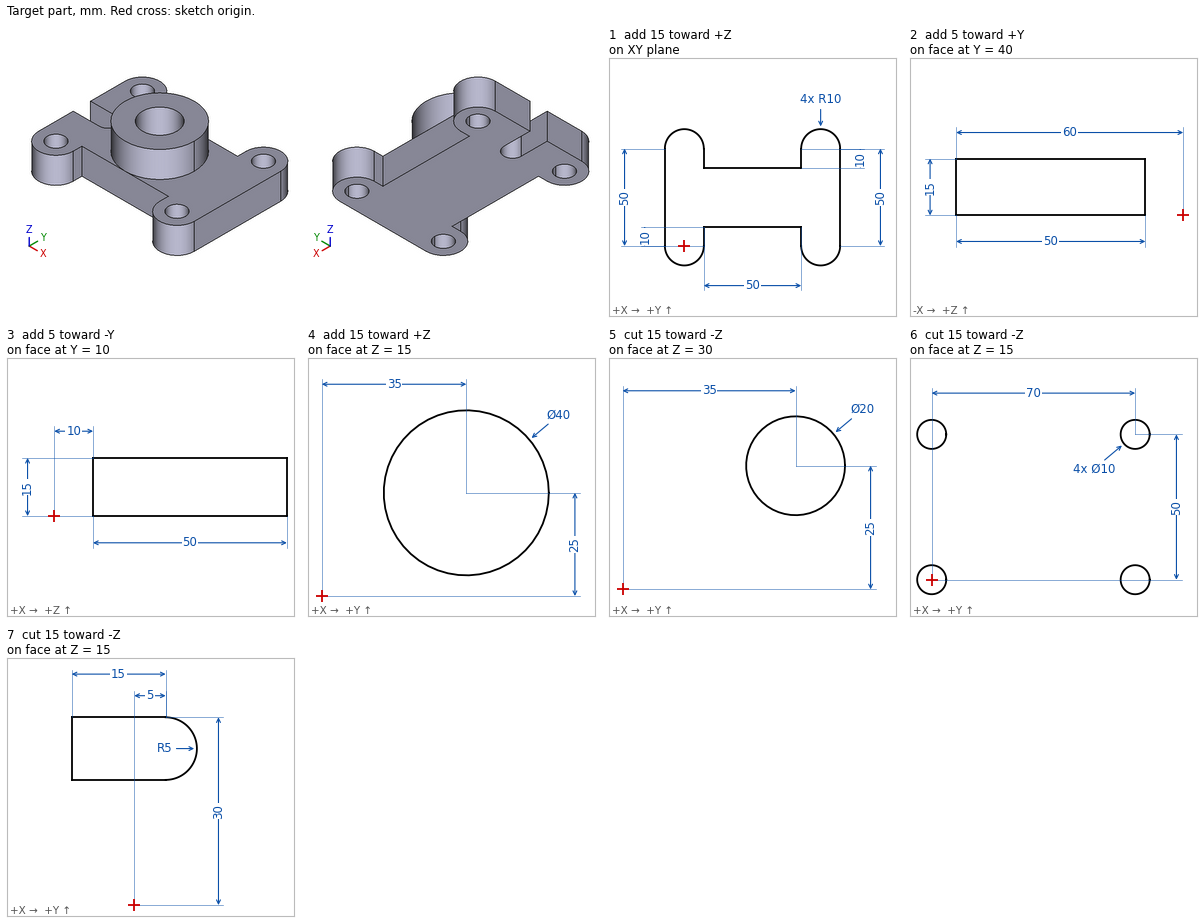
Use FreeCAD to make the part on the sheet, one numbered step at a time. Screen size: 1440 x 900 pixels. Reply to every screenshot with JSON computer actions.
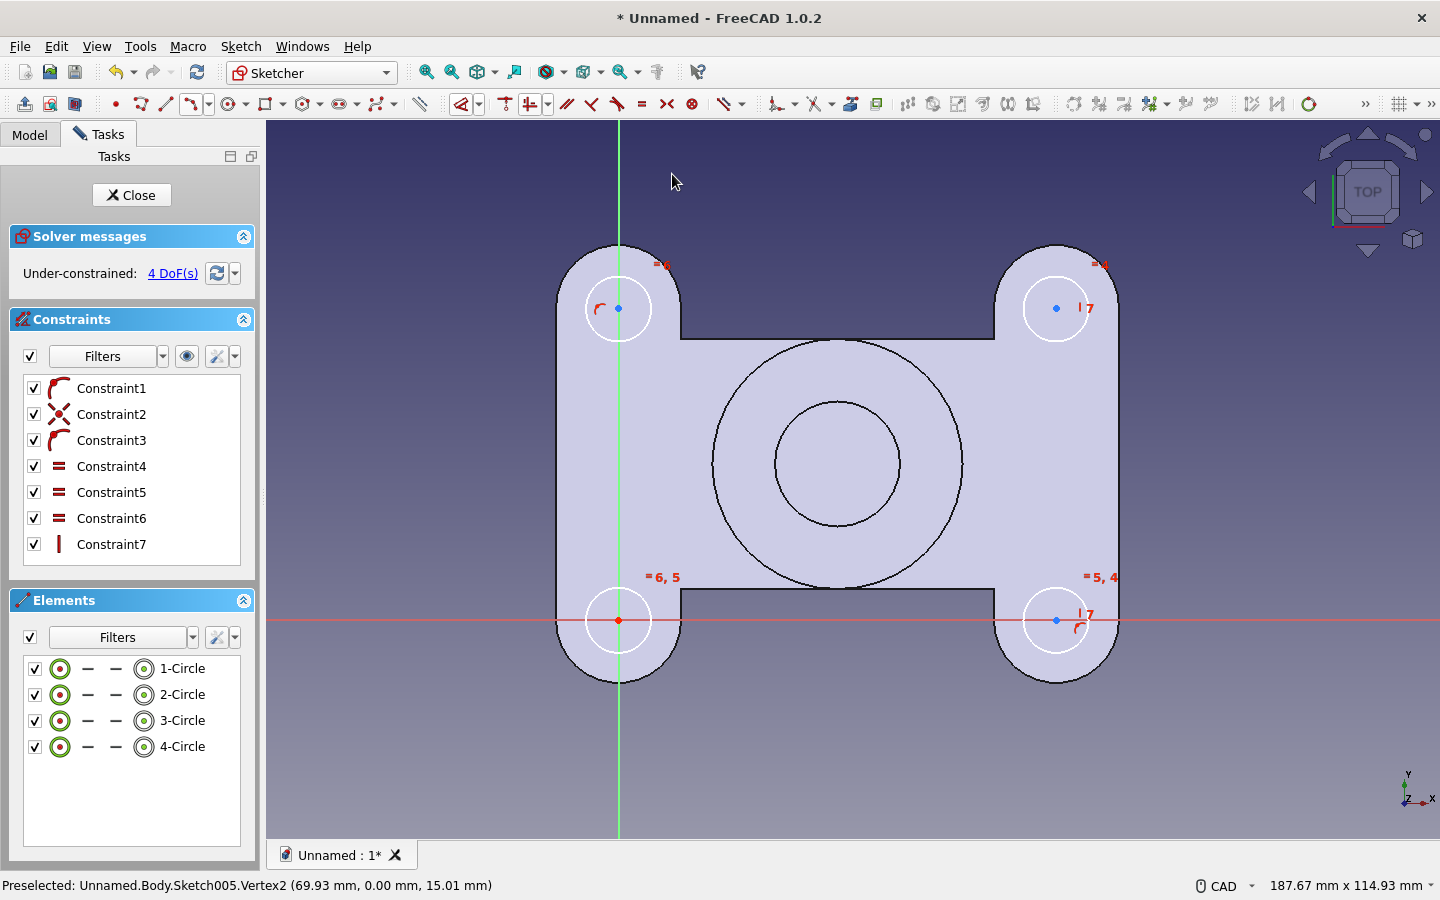
{"action": "left_click", "coordinate": [1056, 309]}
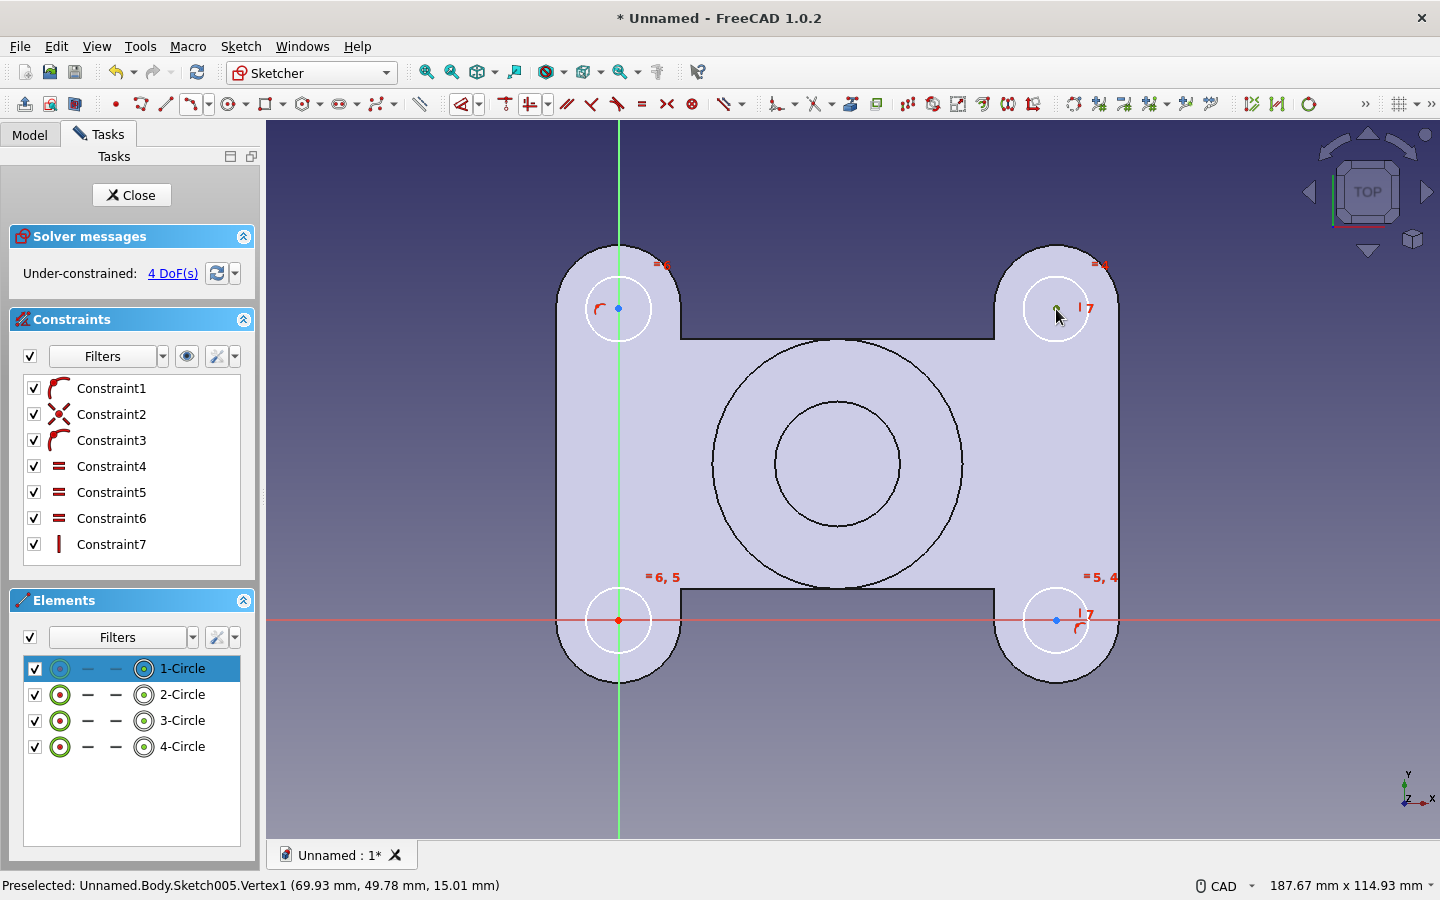
{"action": "left_click", "coordinate": [619, 309]}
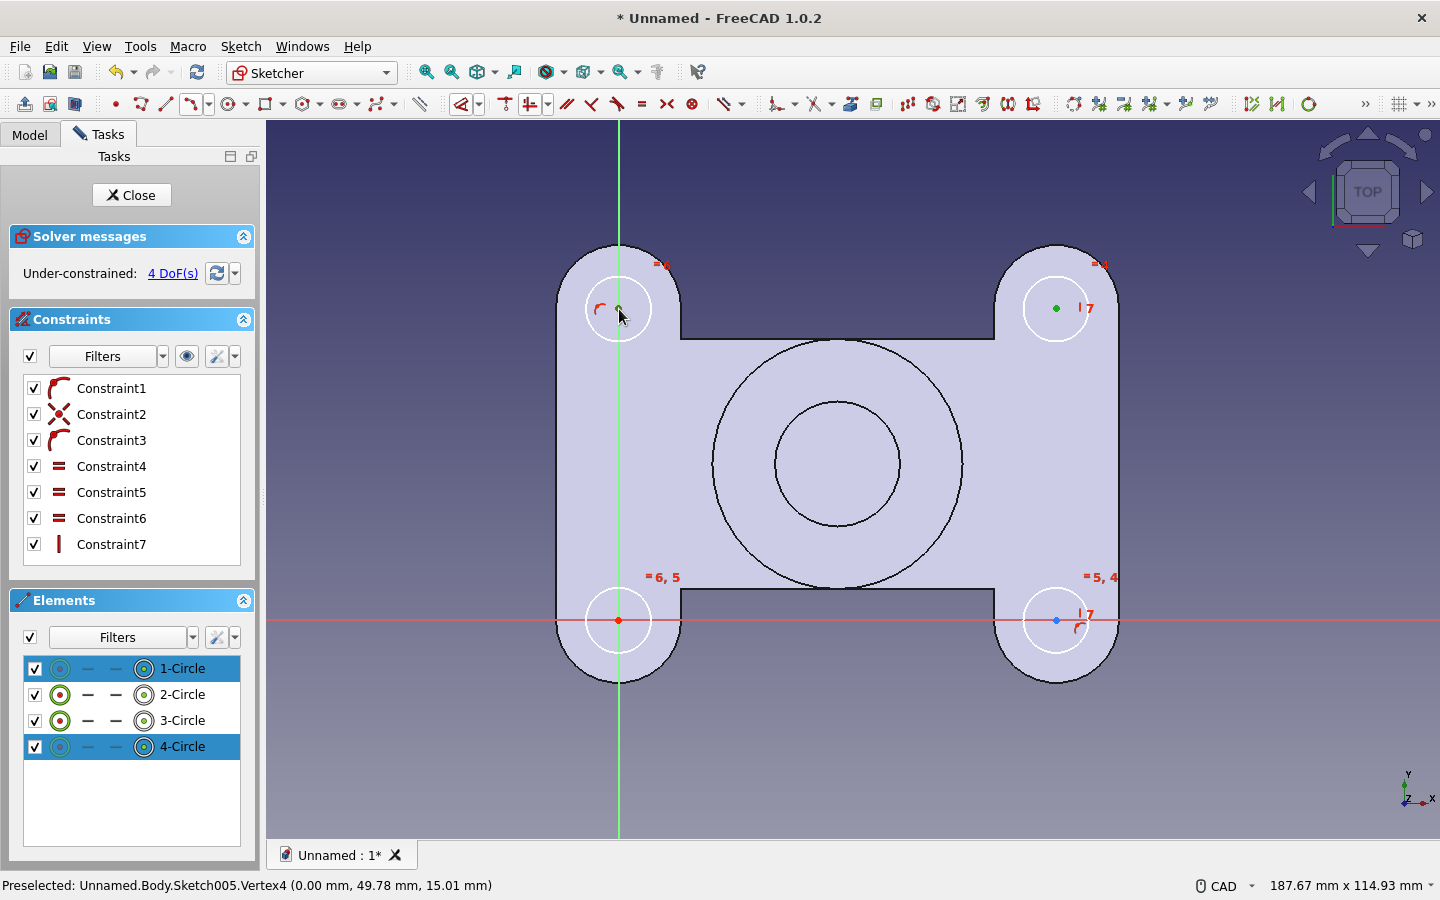
{"action": "left_click", "coordinate": [548, 104]}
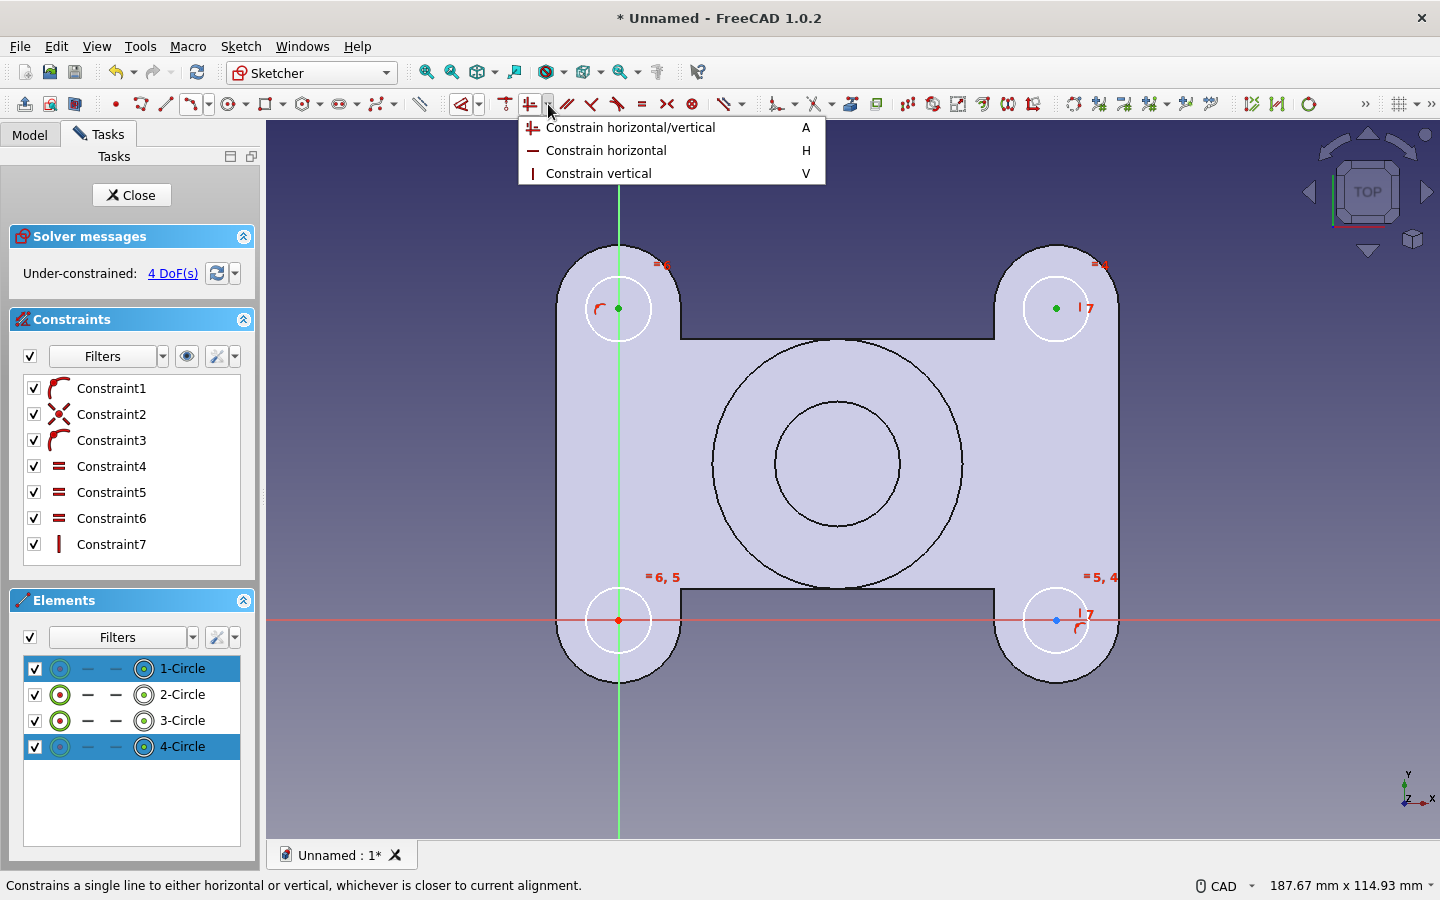
{"action": "left_click", "coordinate": [672, 150]}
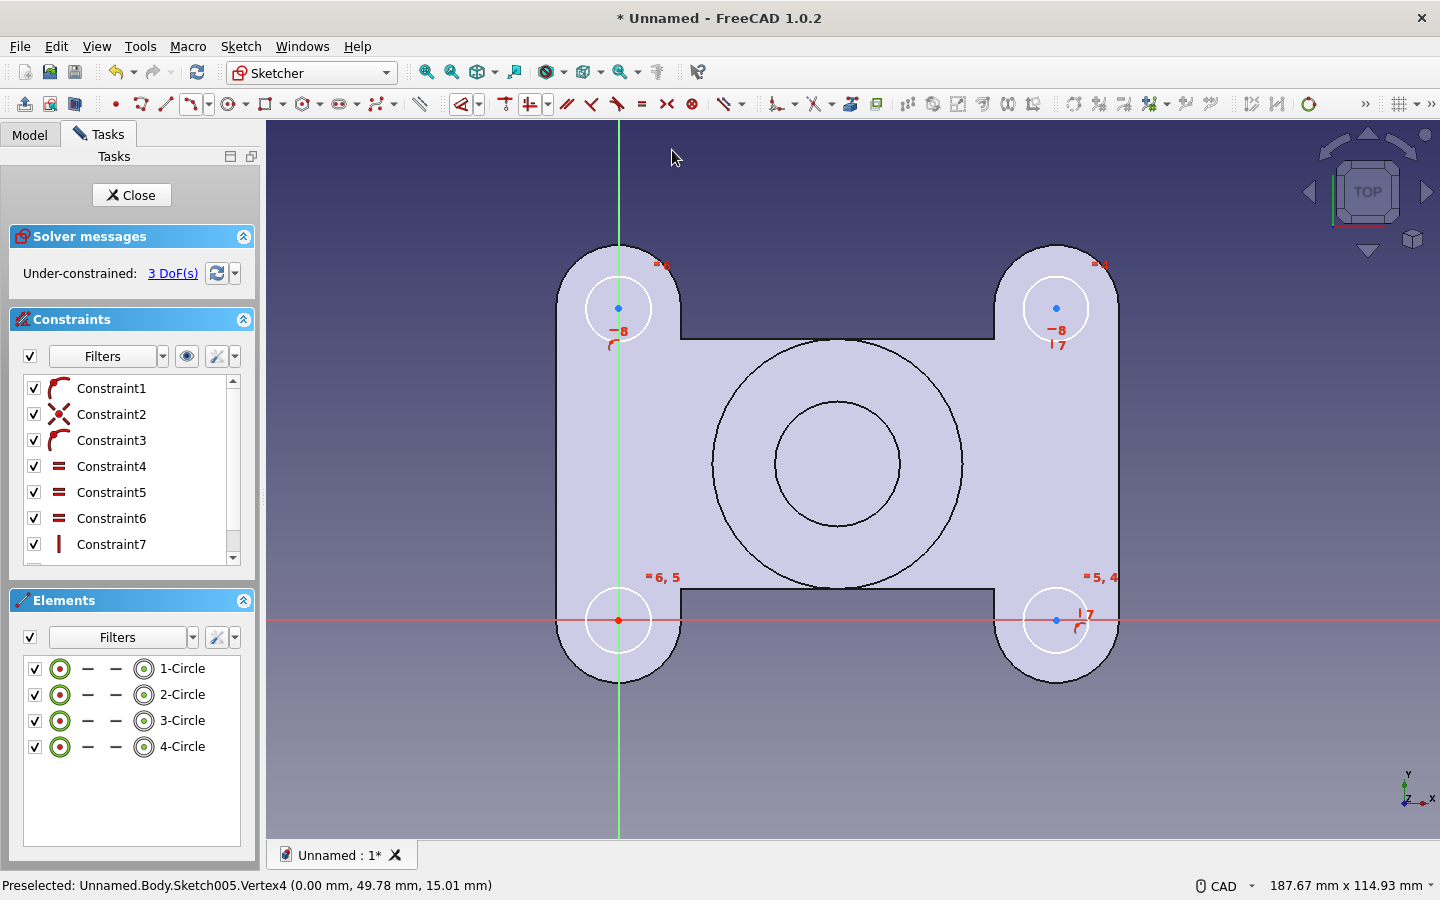
{"action": "left_click", "coordinate": [1079, 286]}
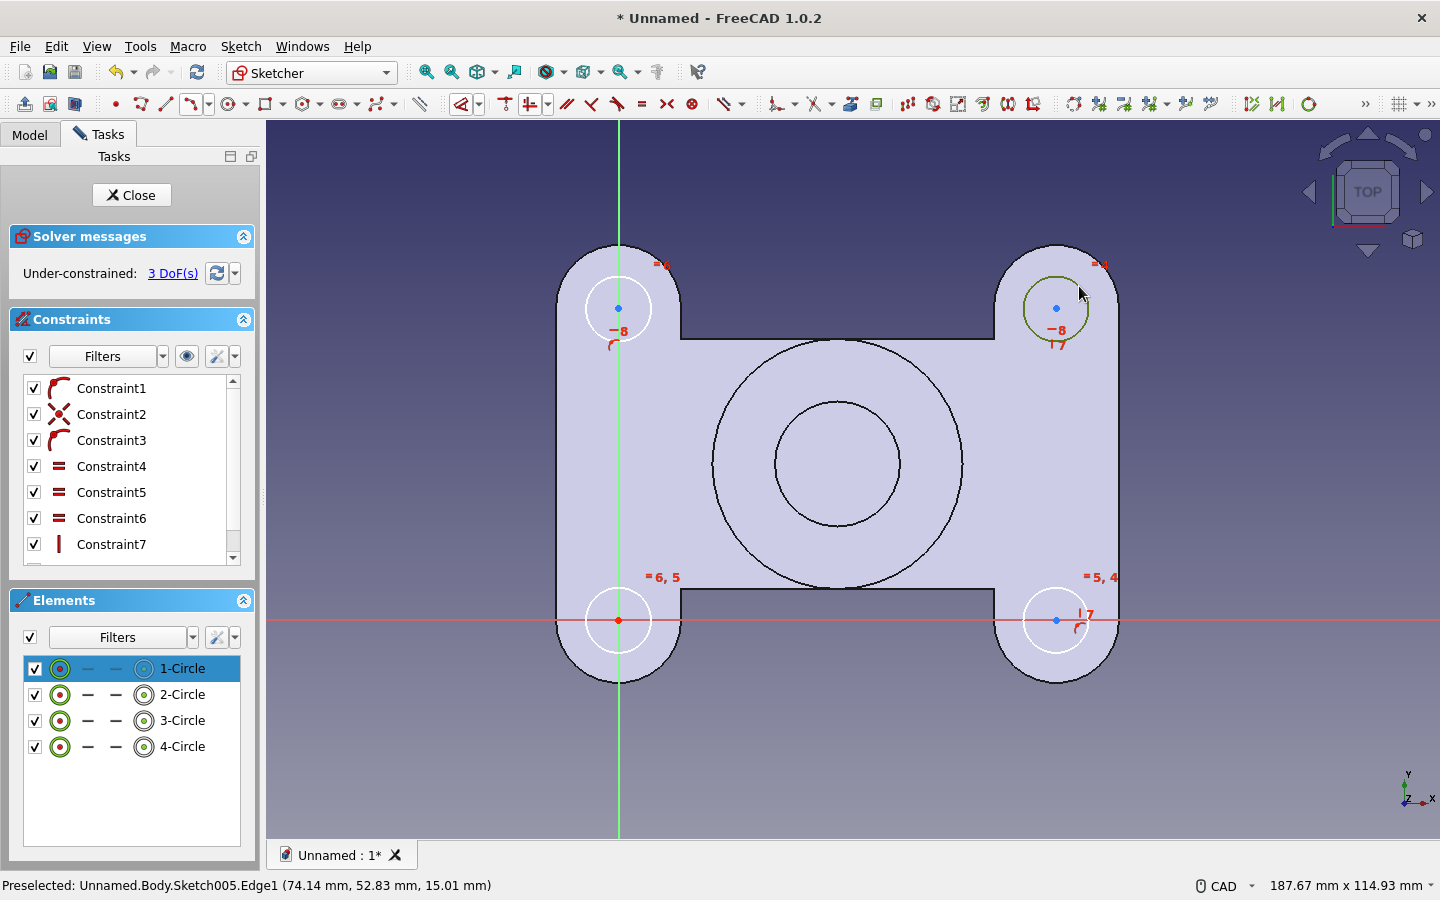
{"action": "key", "text": "k o"}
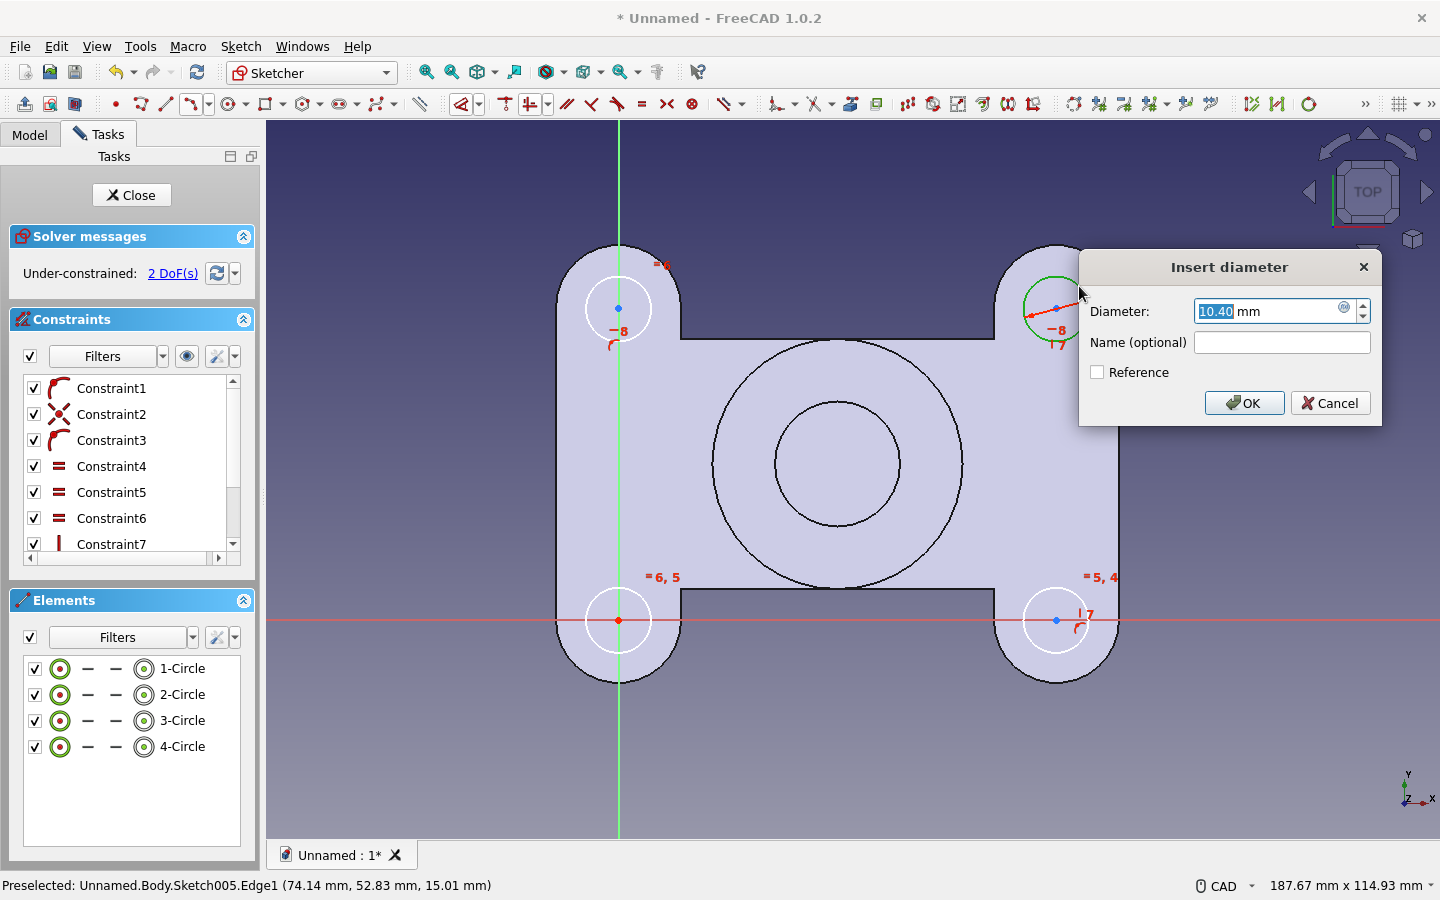
{"action": "type", "text": "10"}
{"action": "key", "text": "Return"}